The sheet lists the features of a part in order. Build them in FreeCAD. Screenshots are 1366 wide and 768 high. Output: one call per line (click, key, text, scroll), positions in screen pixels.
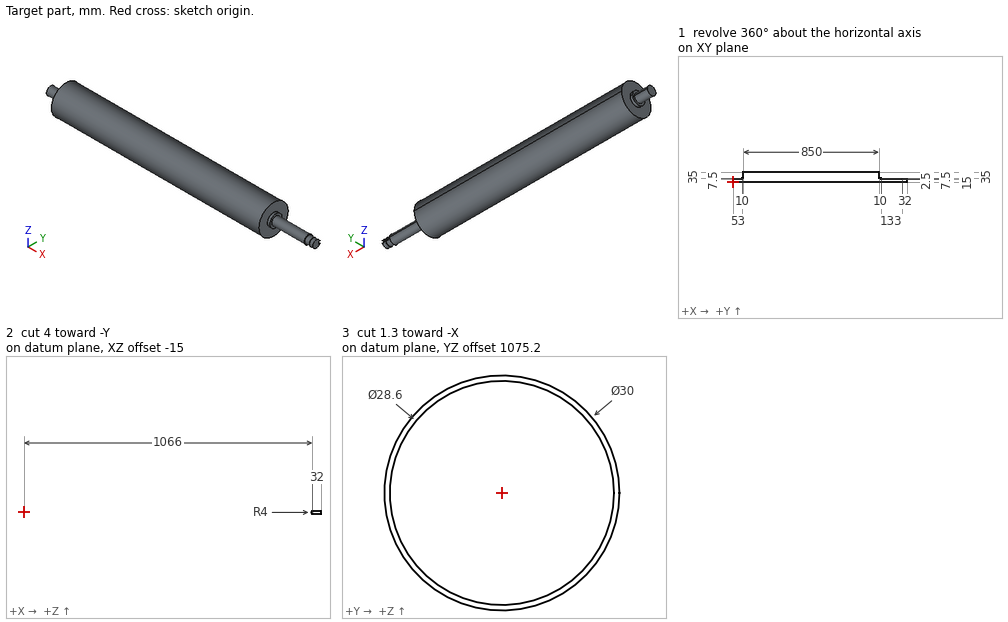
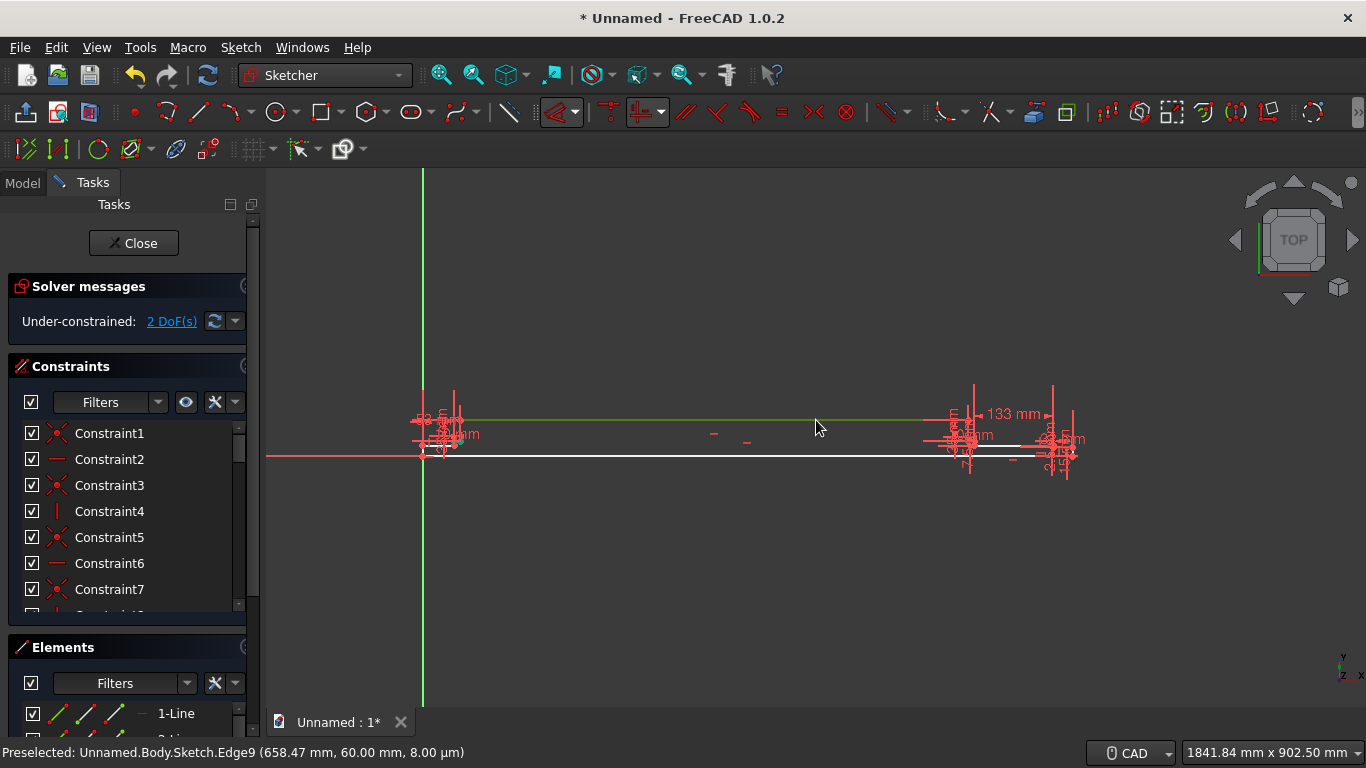
click(578, 112)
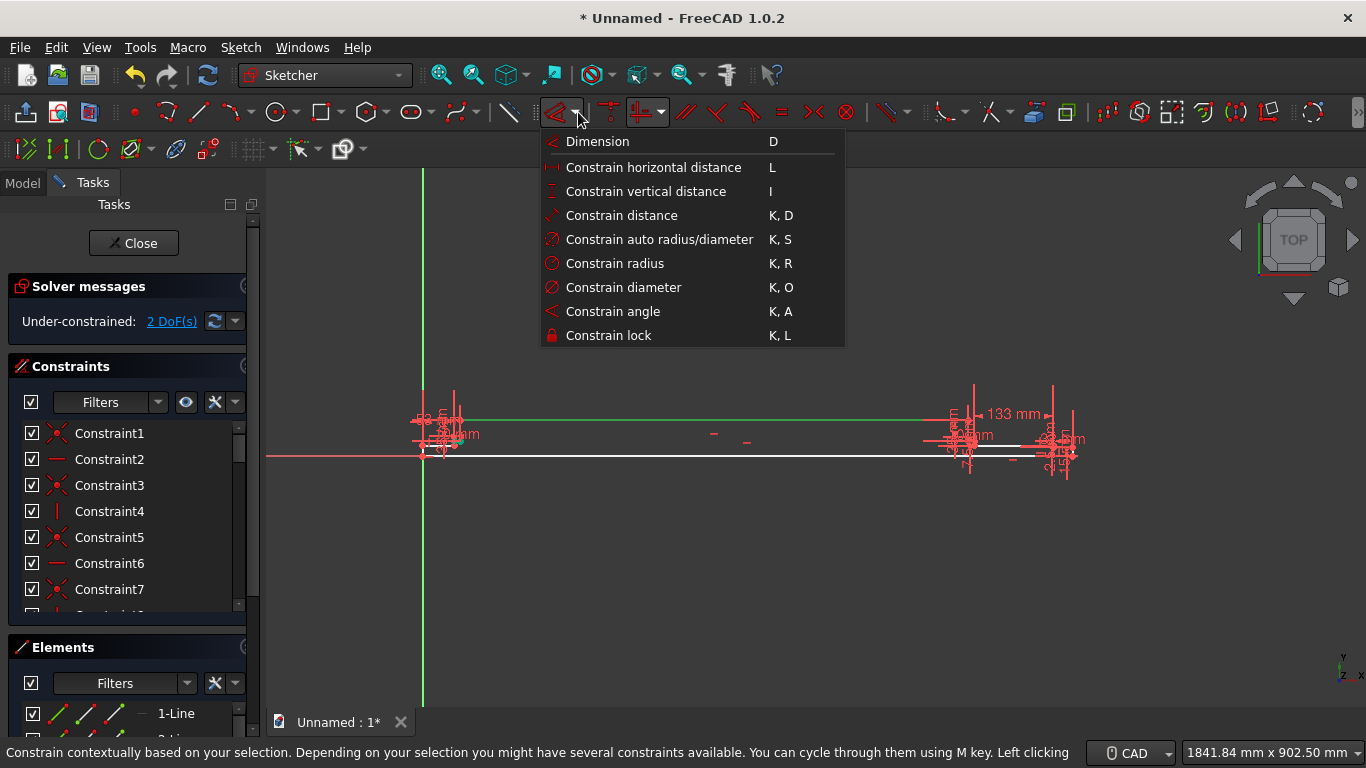
click(693, 167)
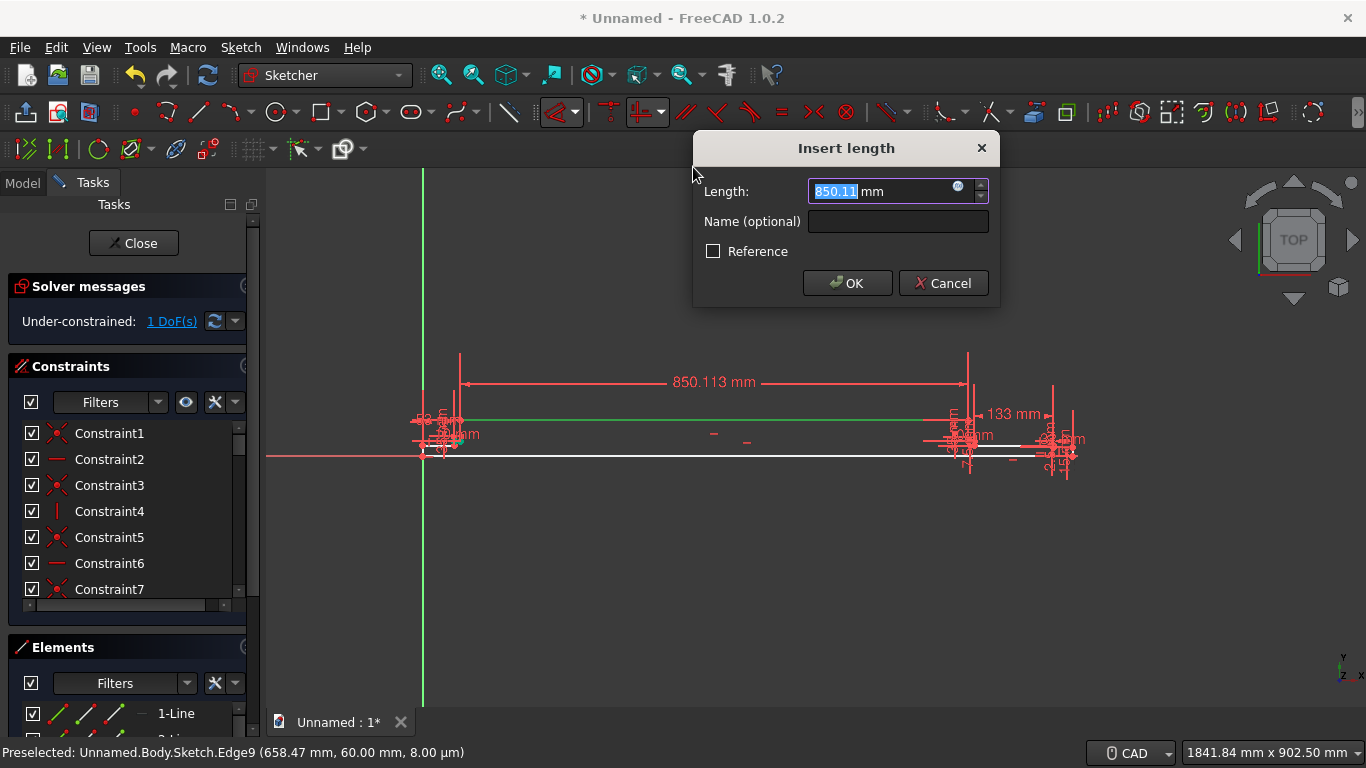
text(850)
key(Return)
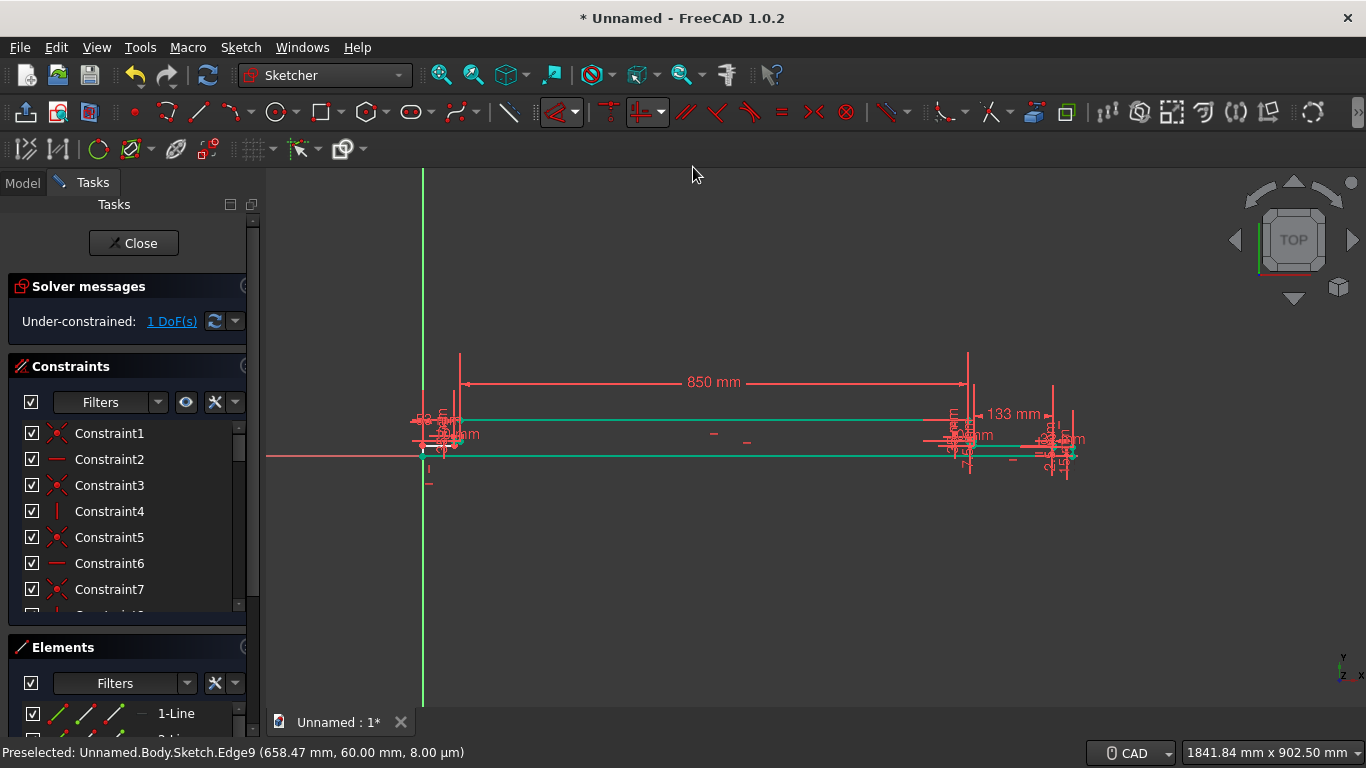
scroll(454, 443, up, 11)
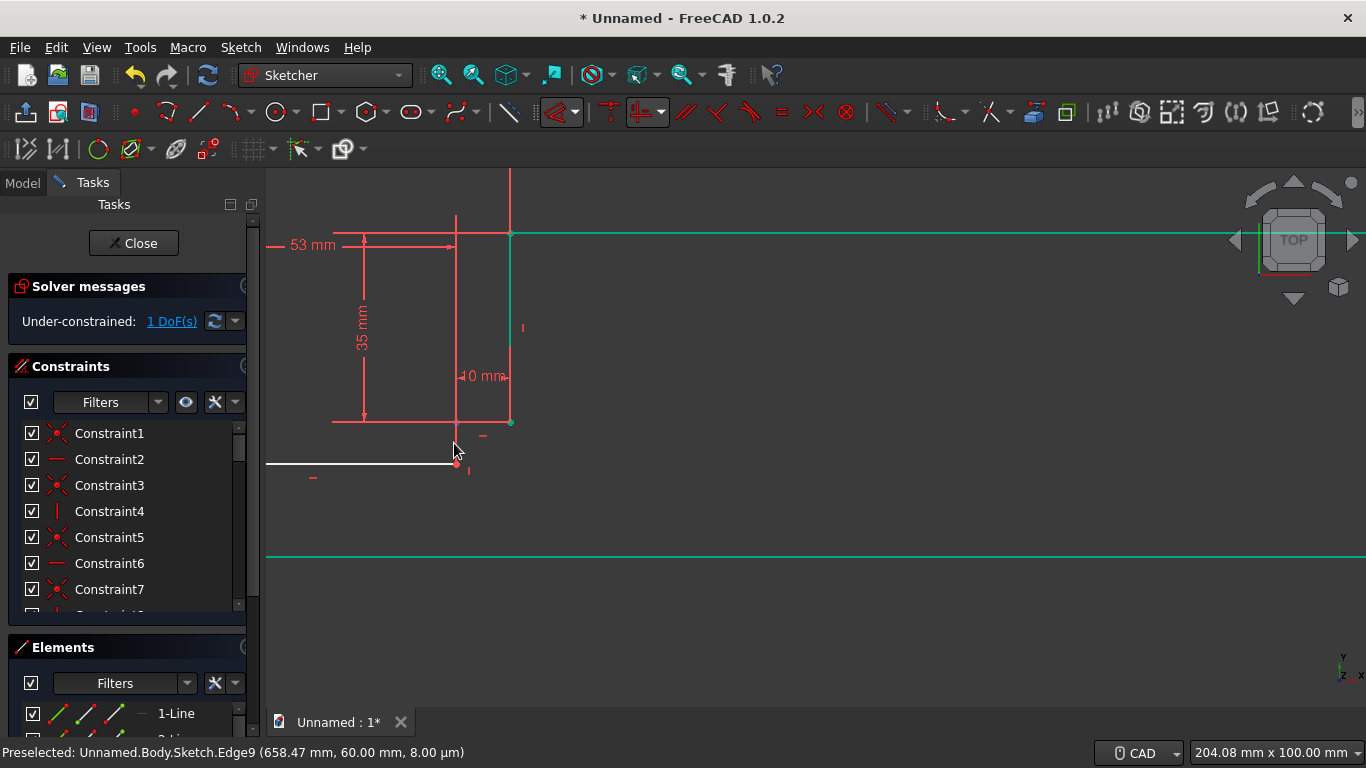
click(456, 443)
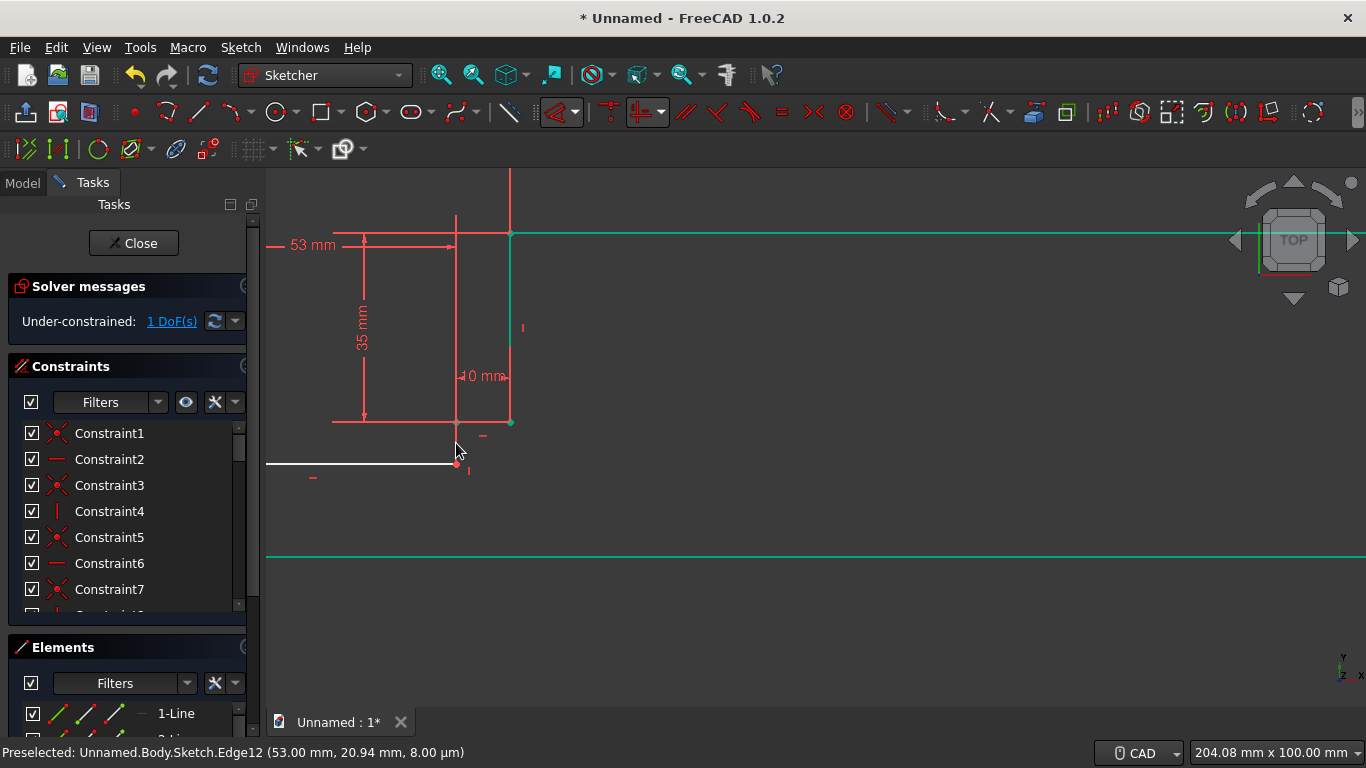
key(i)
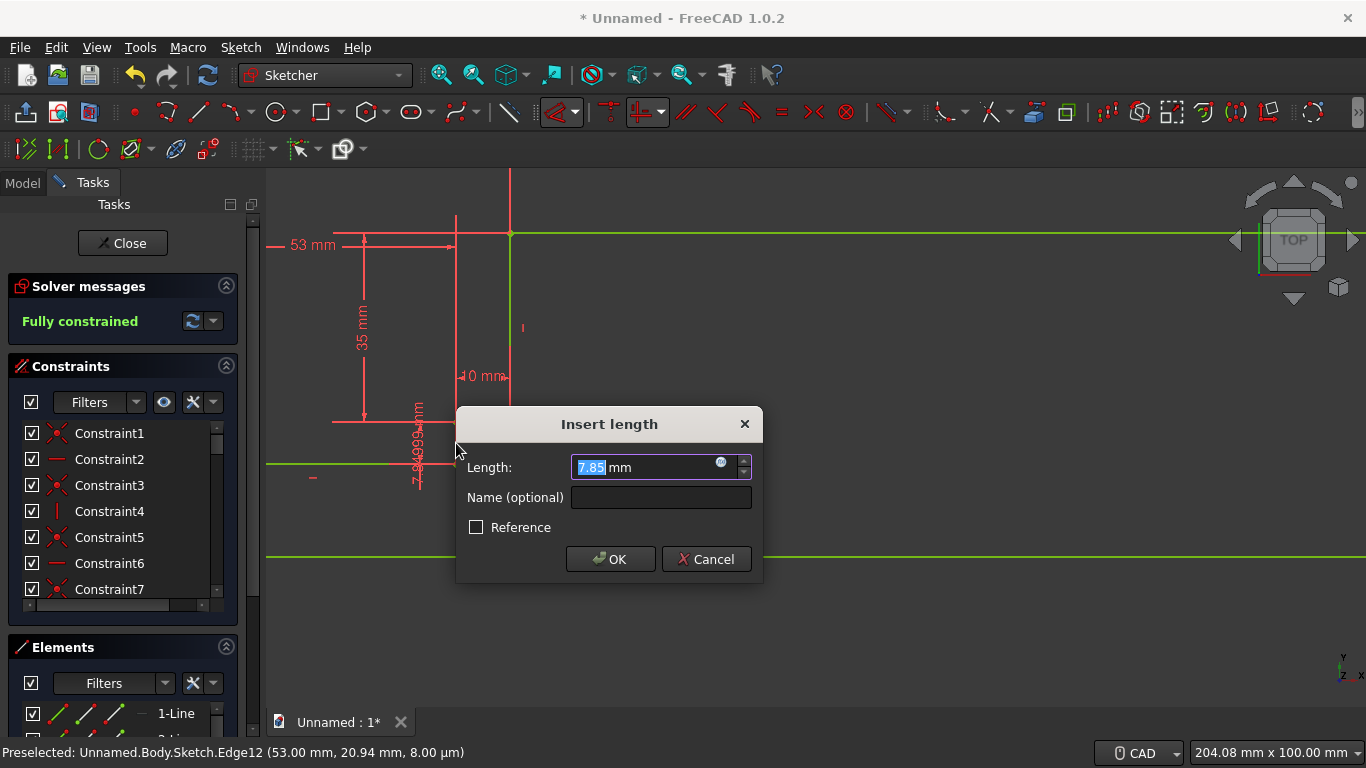
text(7.5)
key(Return)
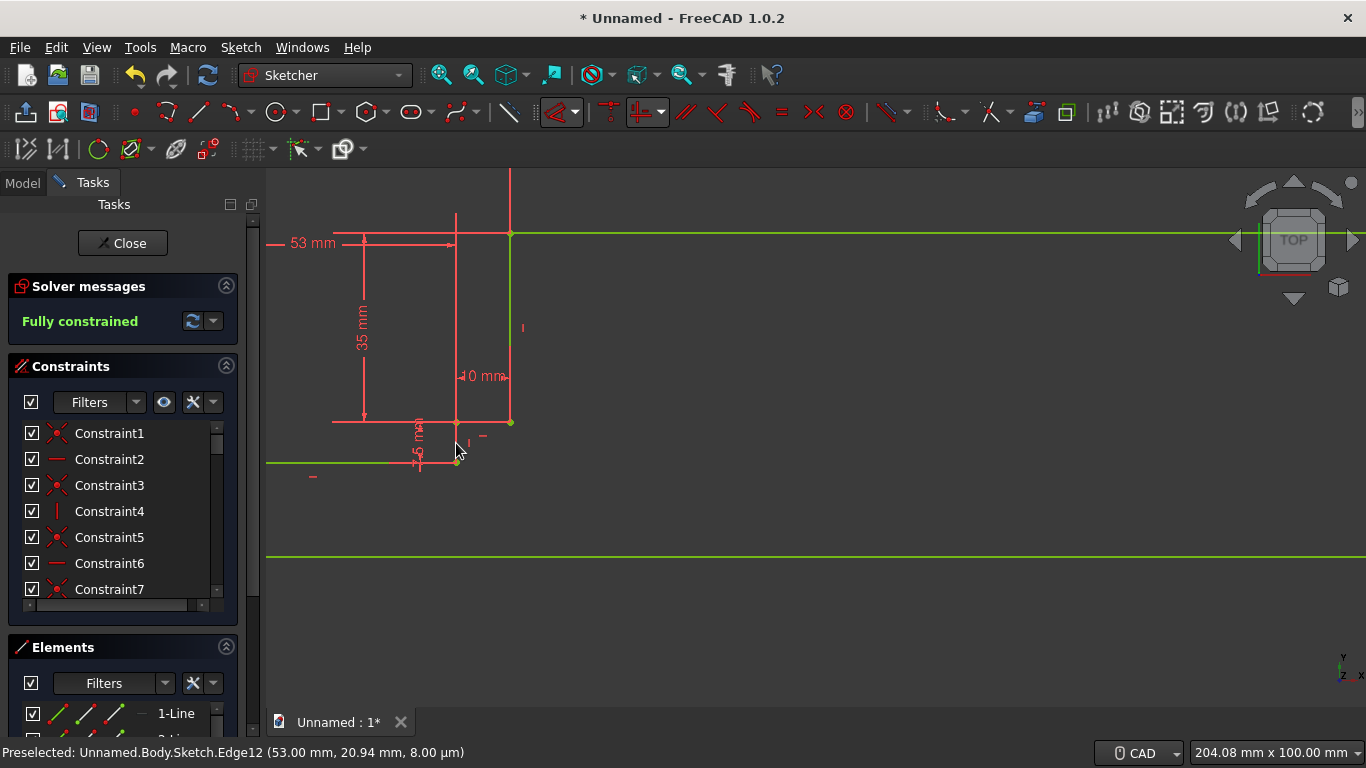
click(123, 243)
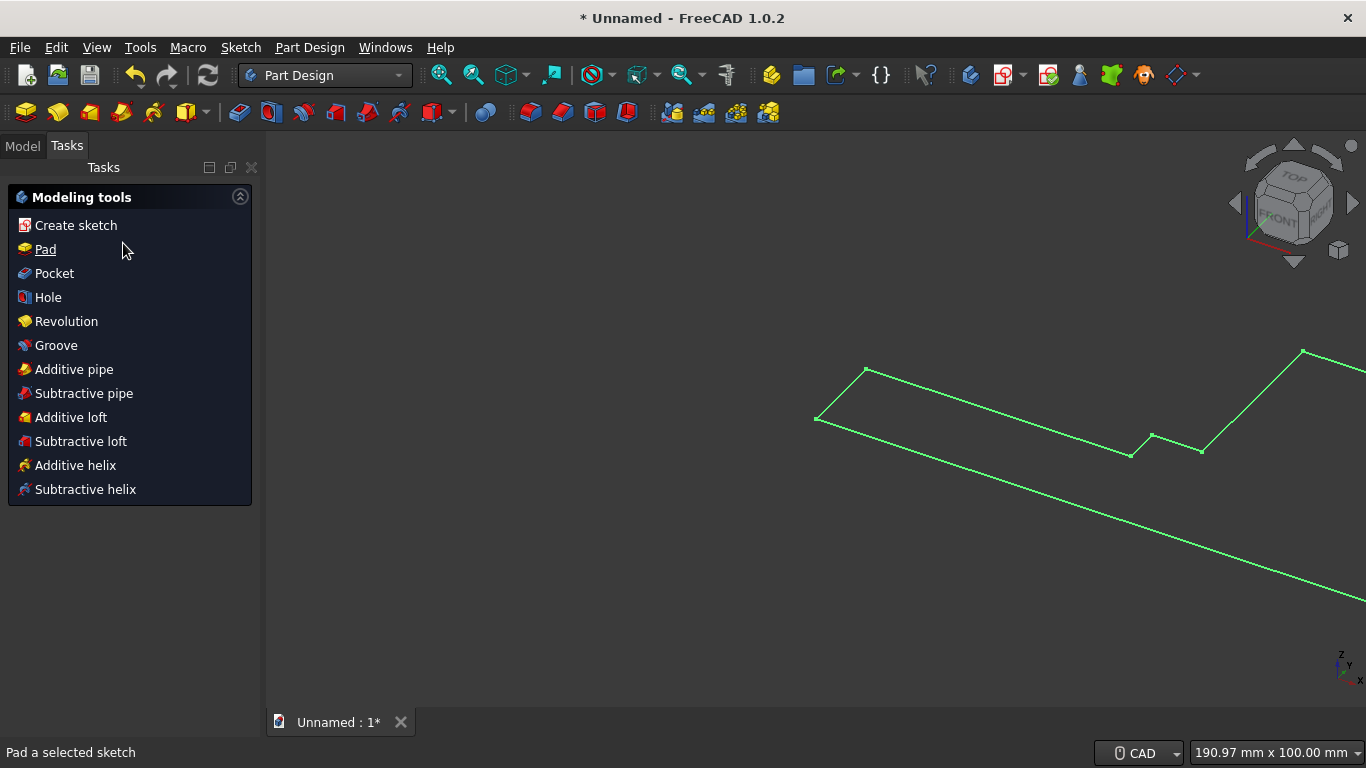
click(58, 112)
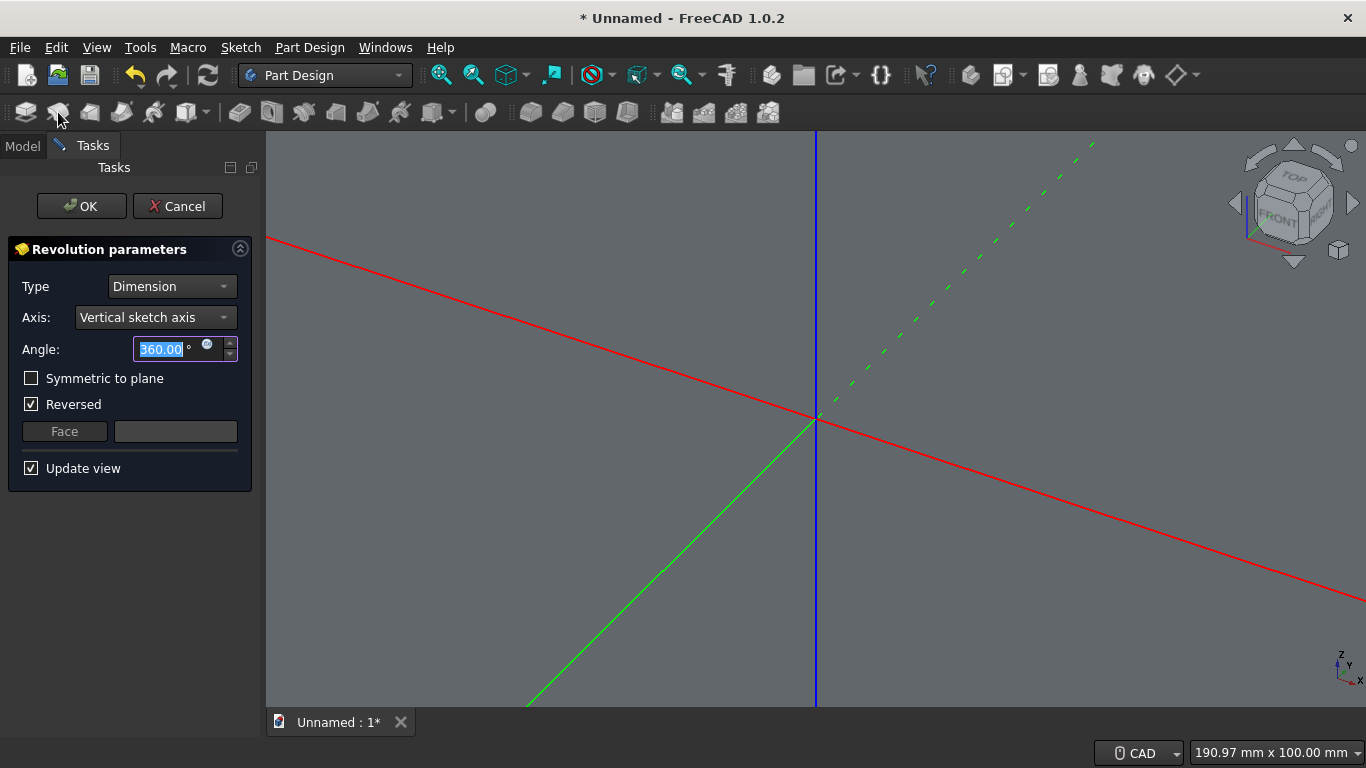
click(156, 318)